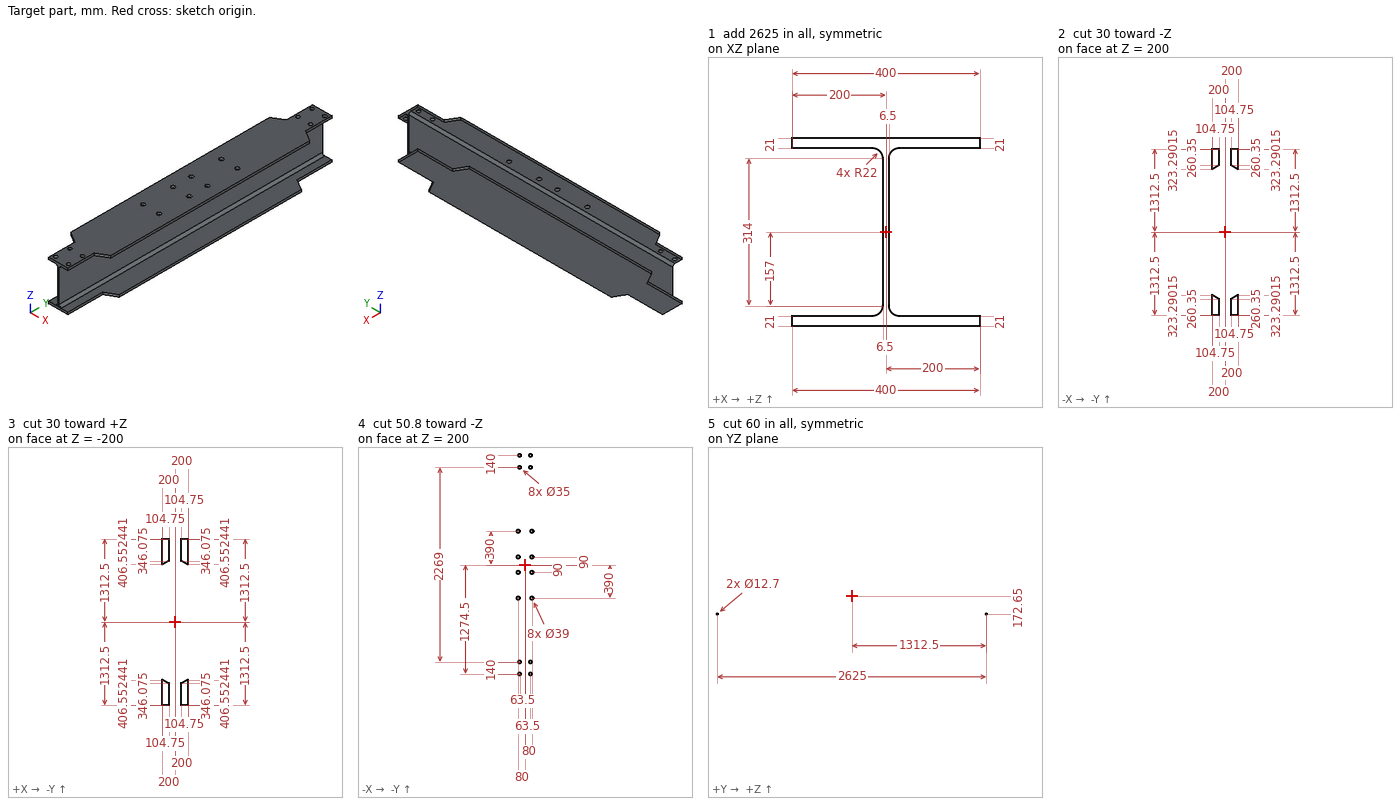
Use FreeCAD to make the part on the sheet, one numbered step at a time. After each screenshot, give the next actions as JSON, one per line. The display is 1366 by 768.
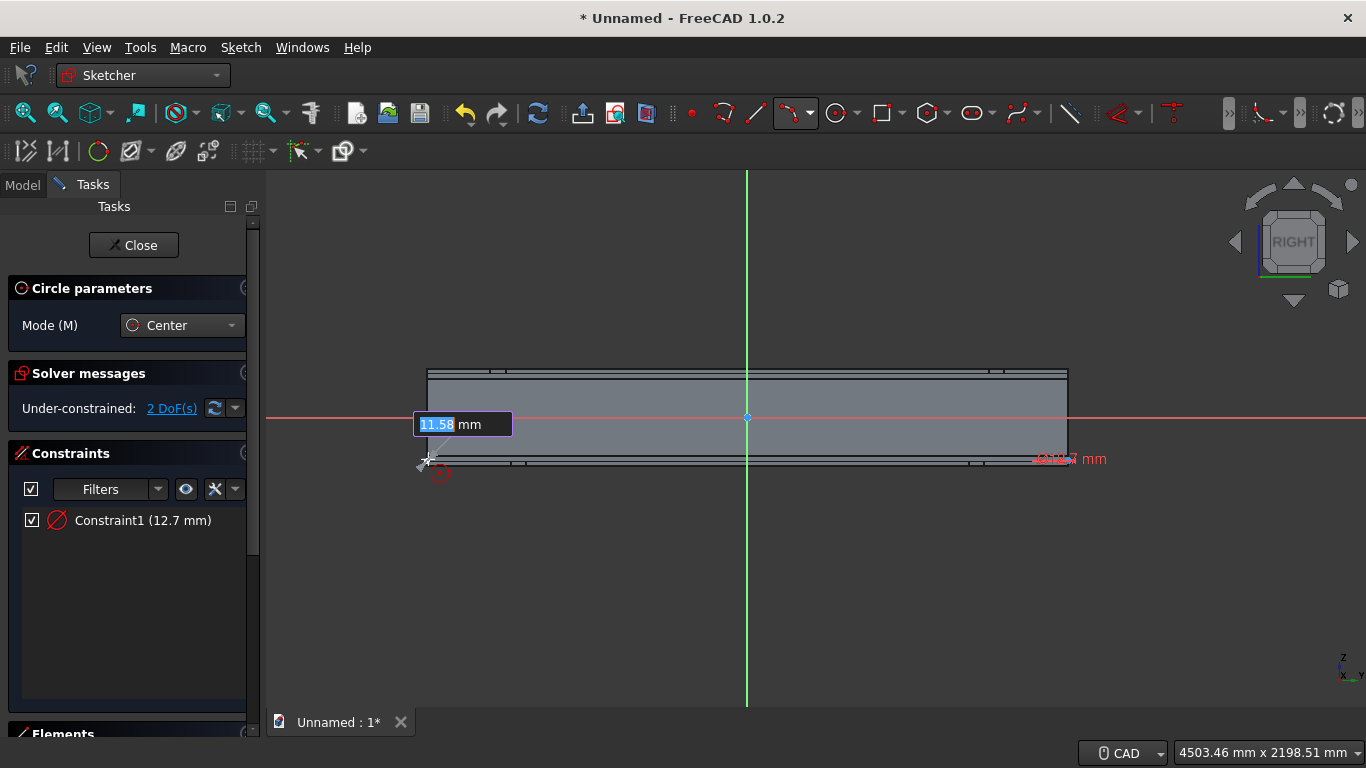
{"action": "type", "text": "12.7"}
{"action": "key", "text": "Return"}
{"action": "key", "text": "Escape"}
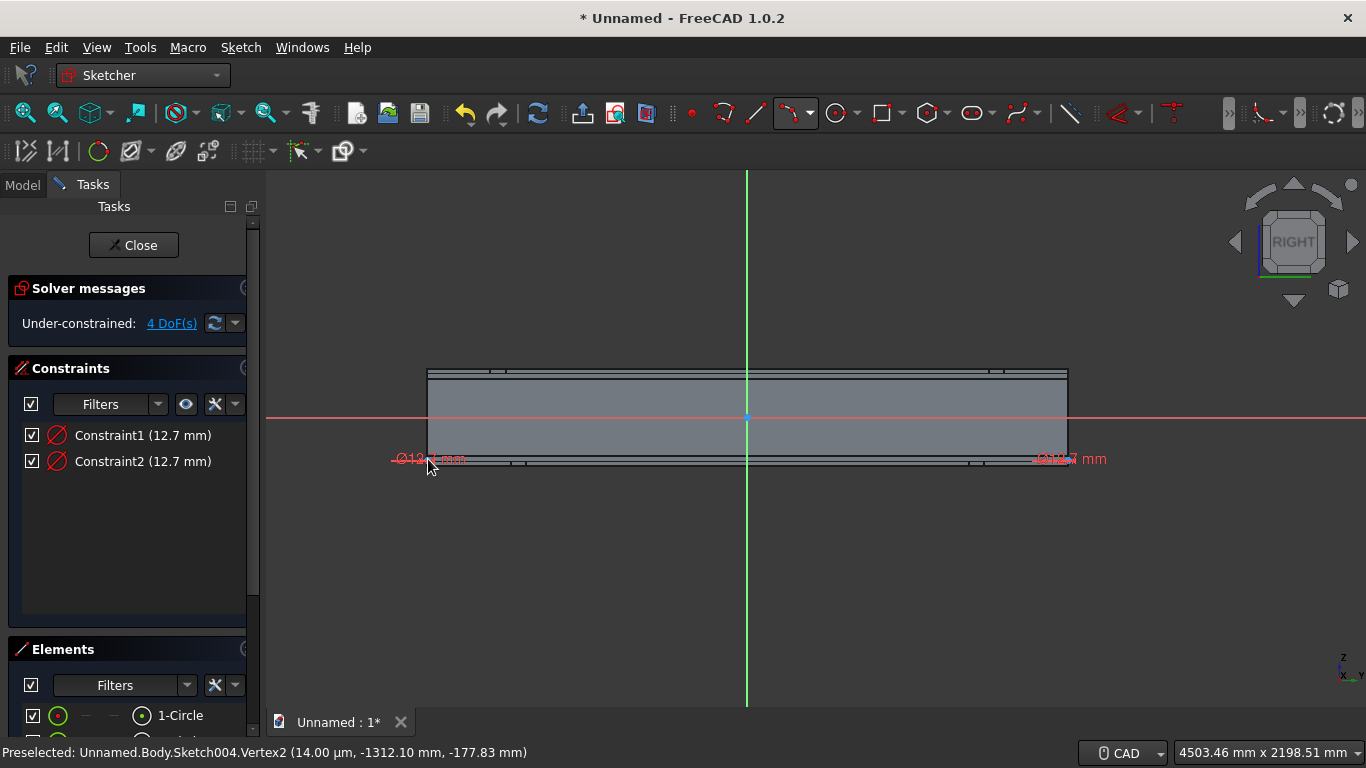
{"action": "left_click", "coordinate": [1068, 461]}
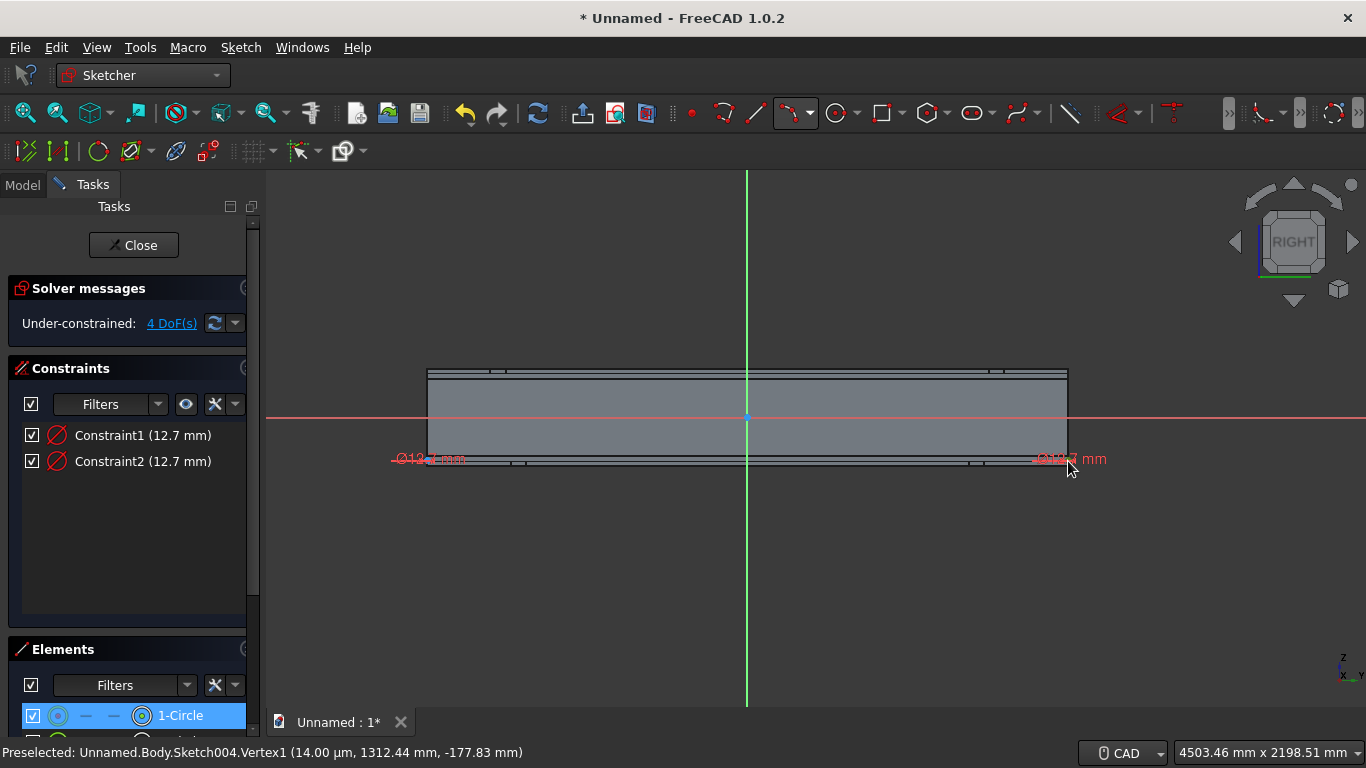
{"action": "left_click", "coordinate": [427, 461]}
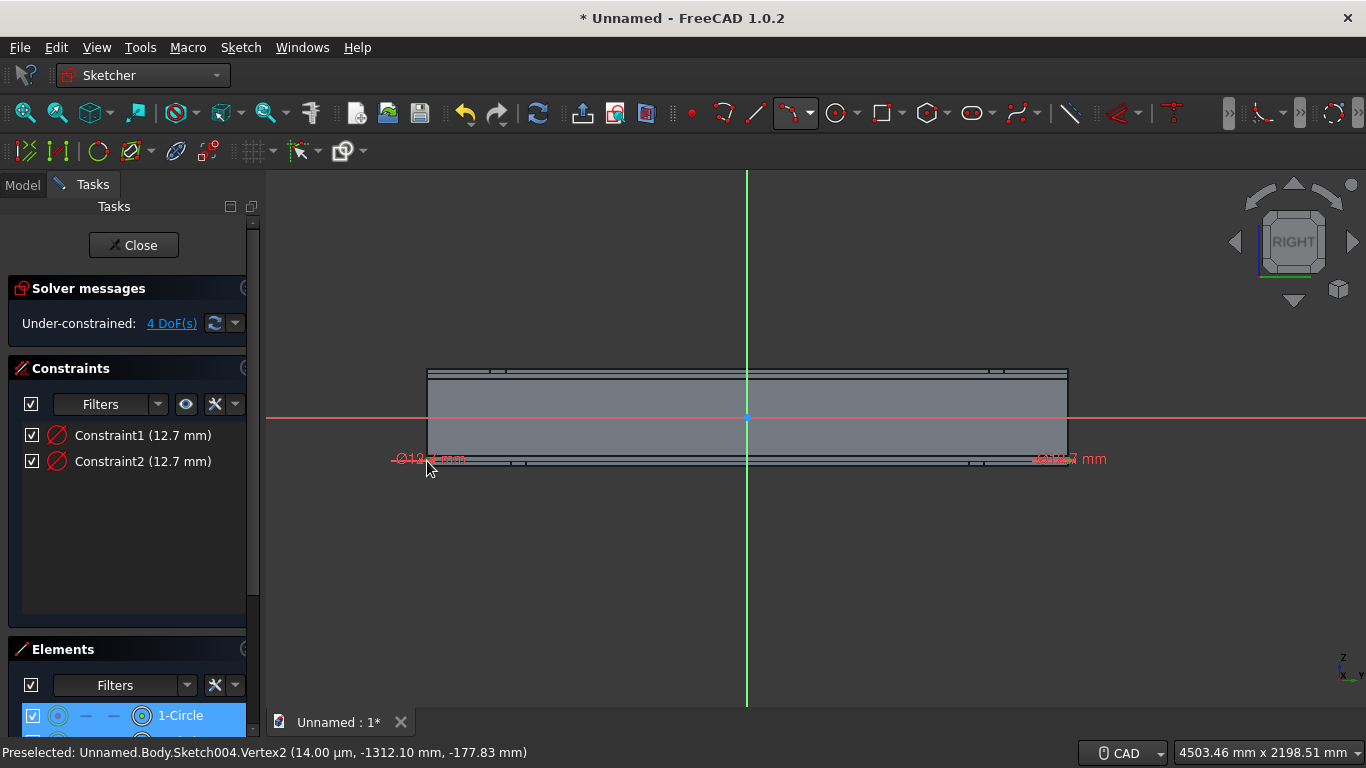
{"action": "key", "text": "h"}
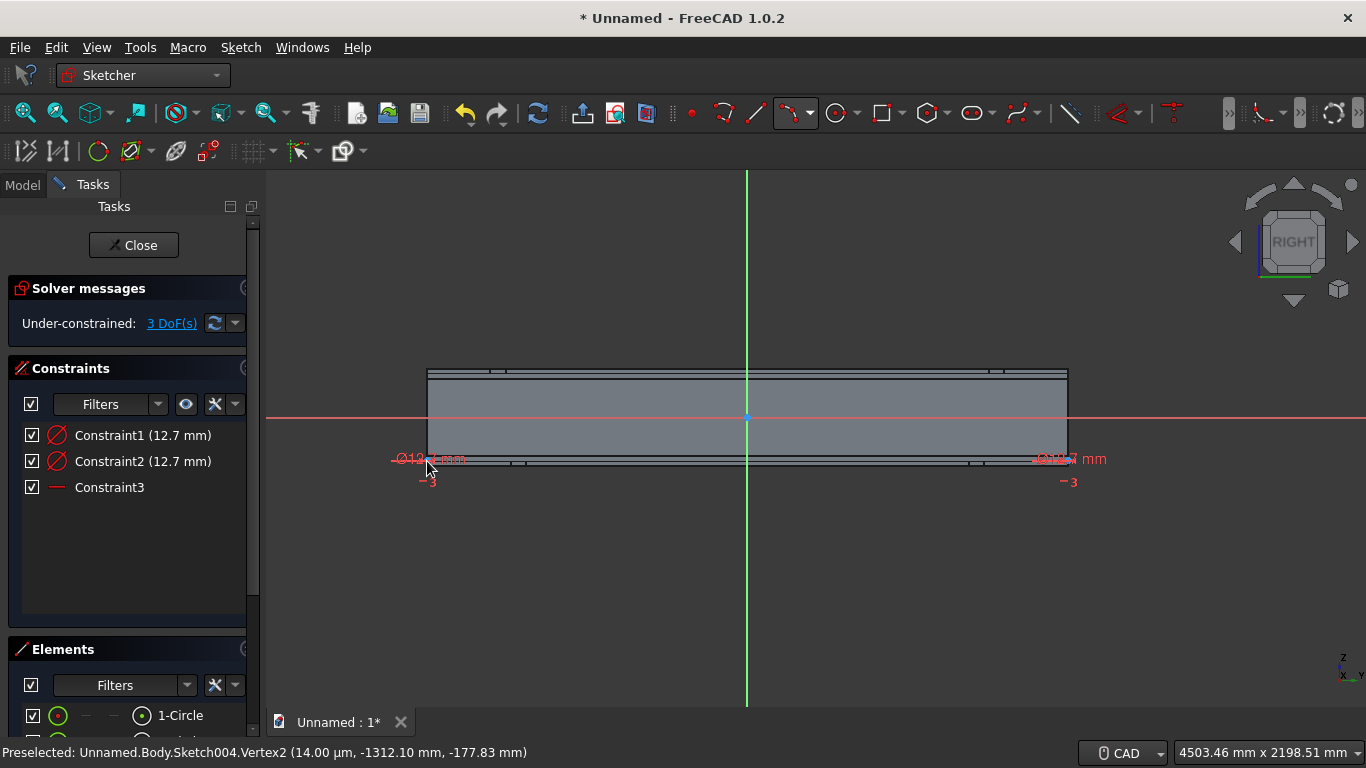
{"action": "left_click", "coordinate": [1118, 114]}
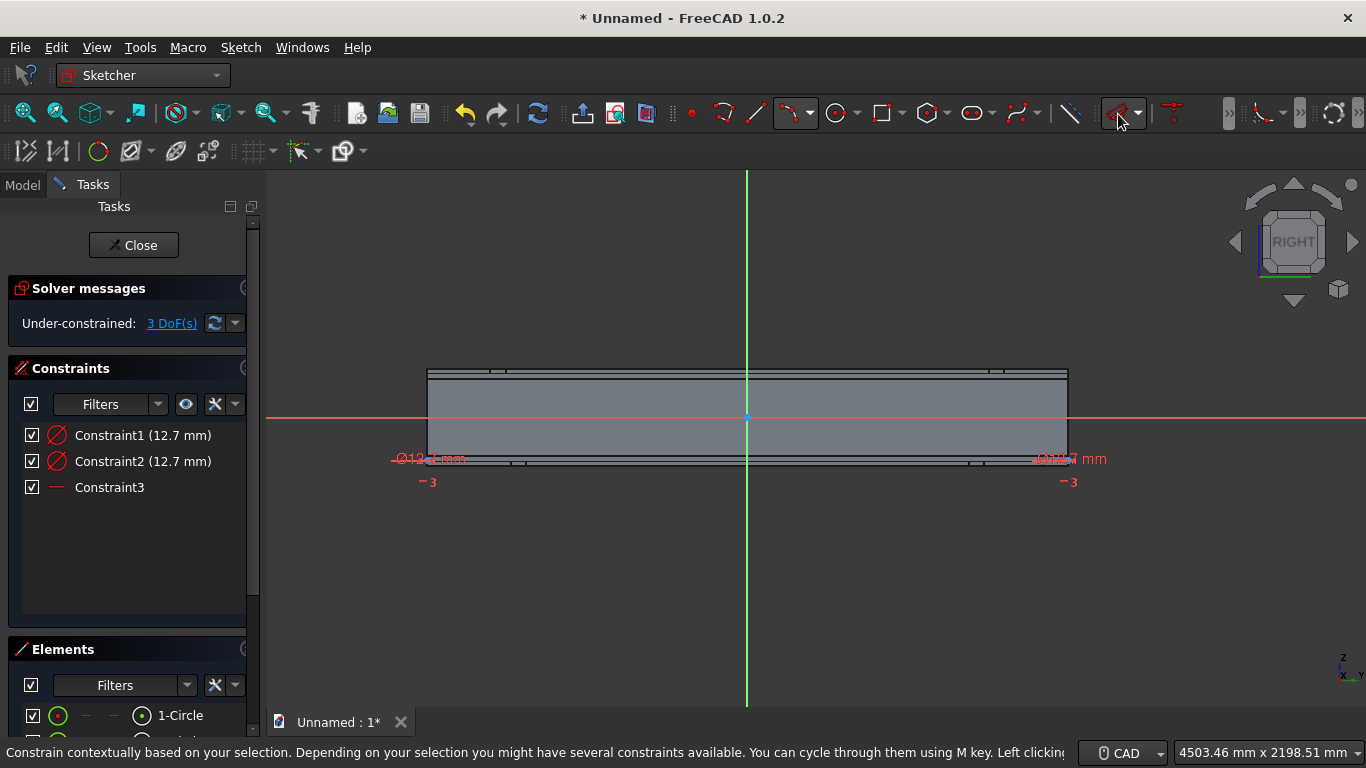
{"action": "left_click", "coordinate": [1068, 461]}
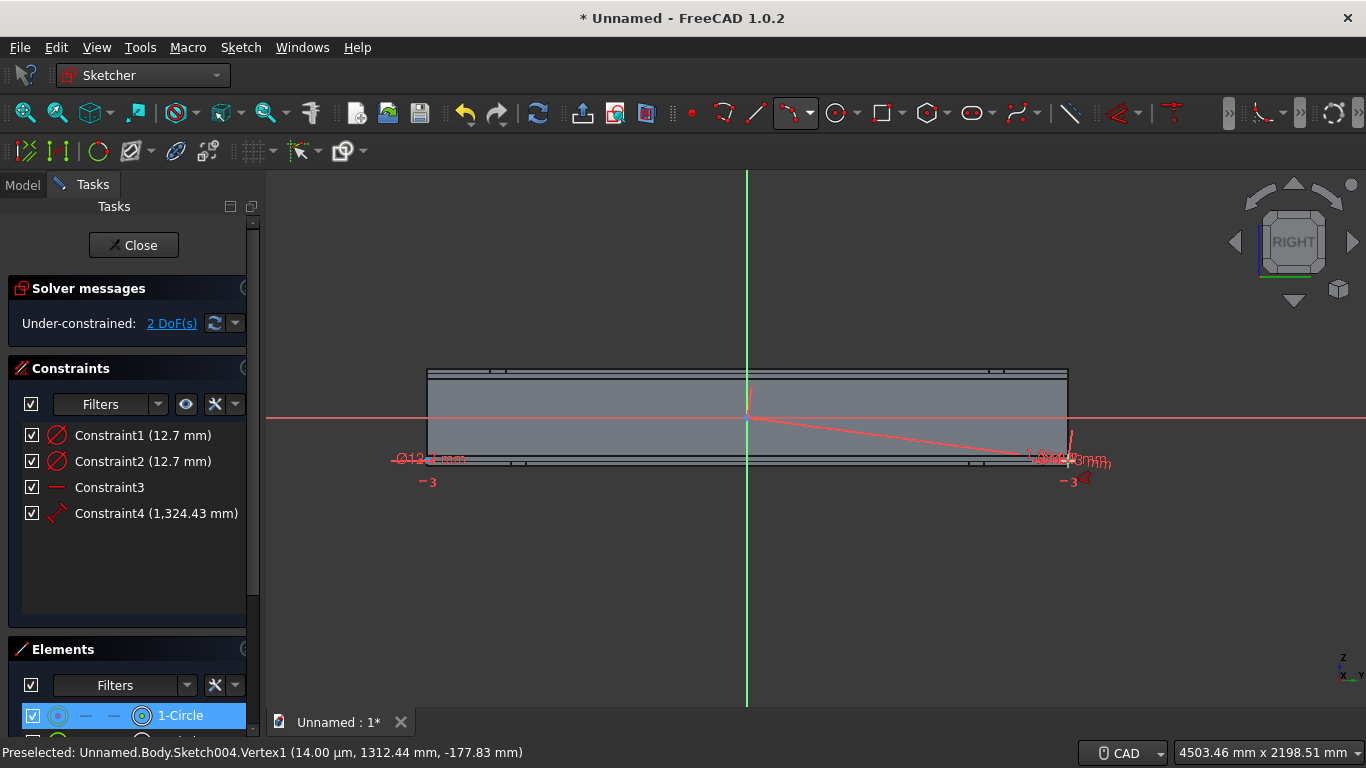
{"action": "left_click", "coordinate": [427, 461]}
{"action": "left_click", "coordinate": [600, 495]}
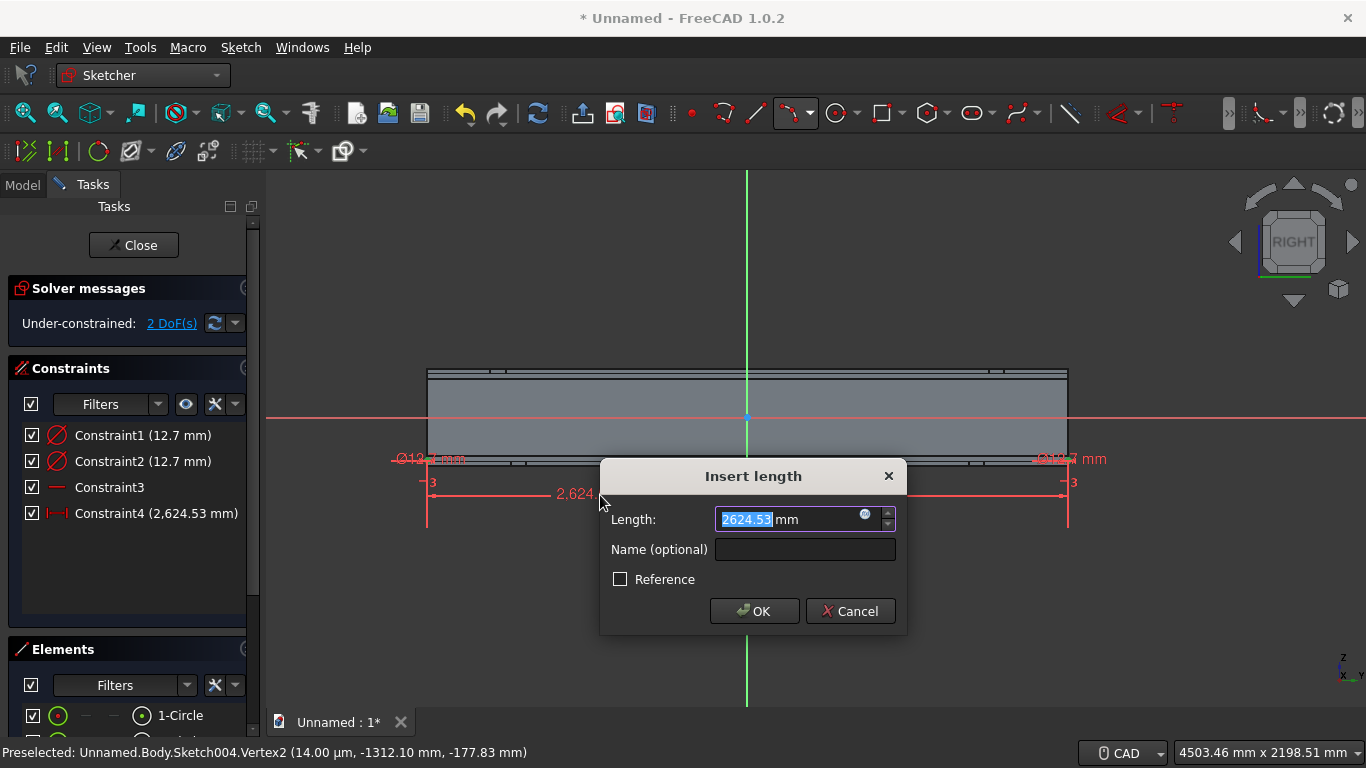
{"action": "type", "text": "2625"}
{"action": "key", "text": "Return"}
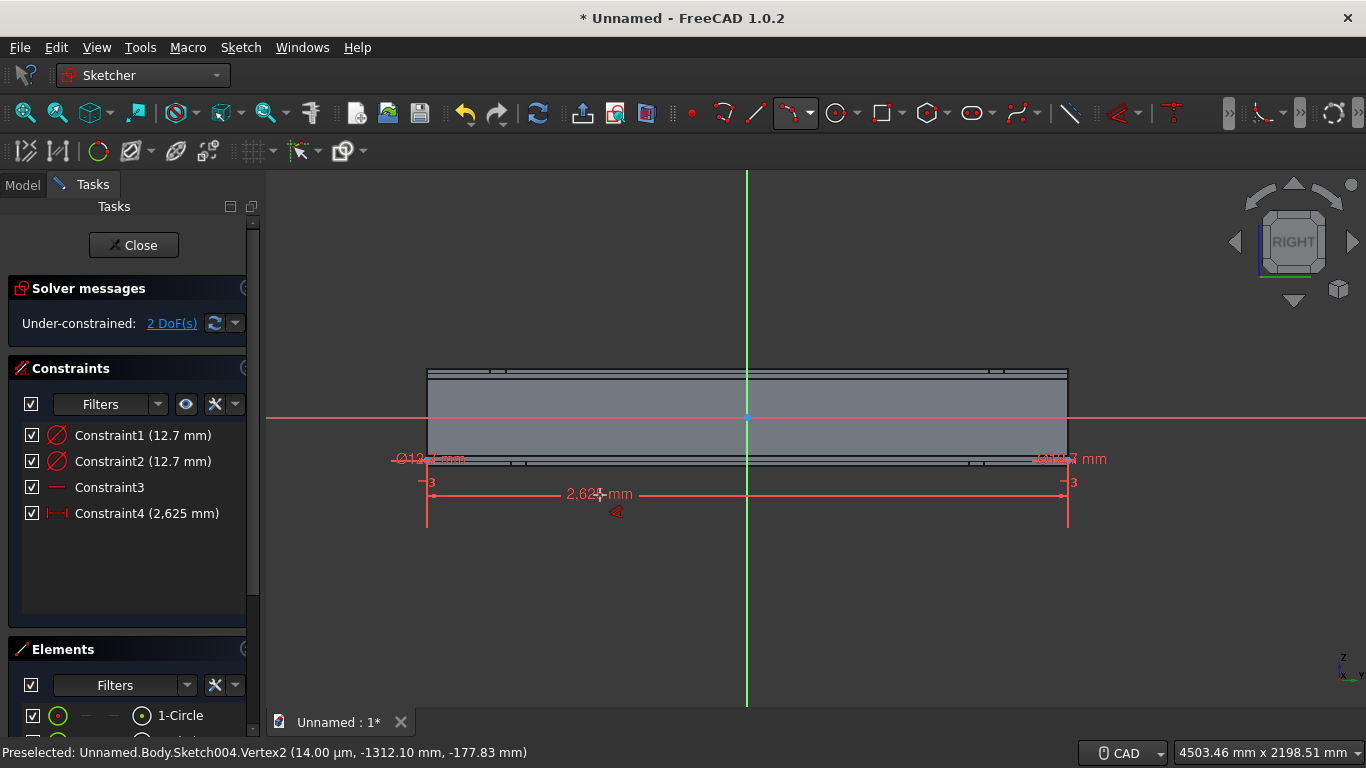
{"action": "left_click", "coordinate": [1068, 461]}
{"action": "left_click", "coordinate": [908, 384]}